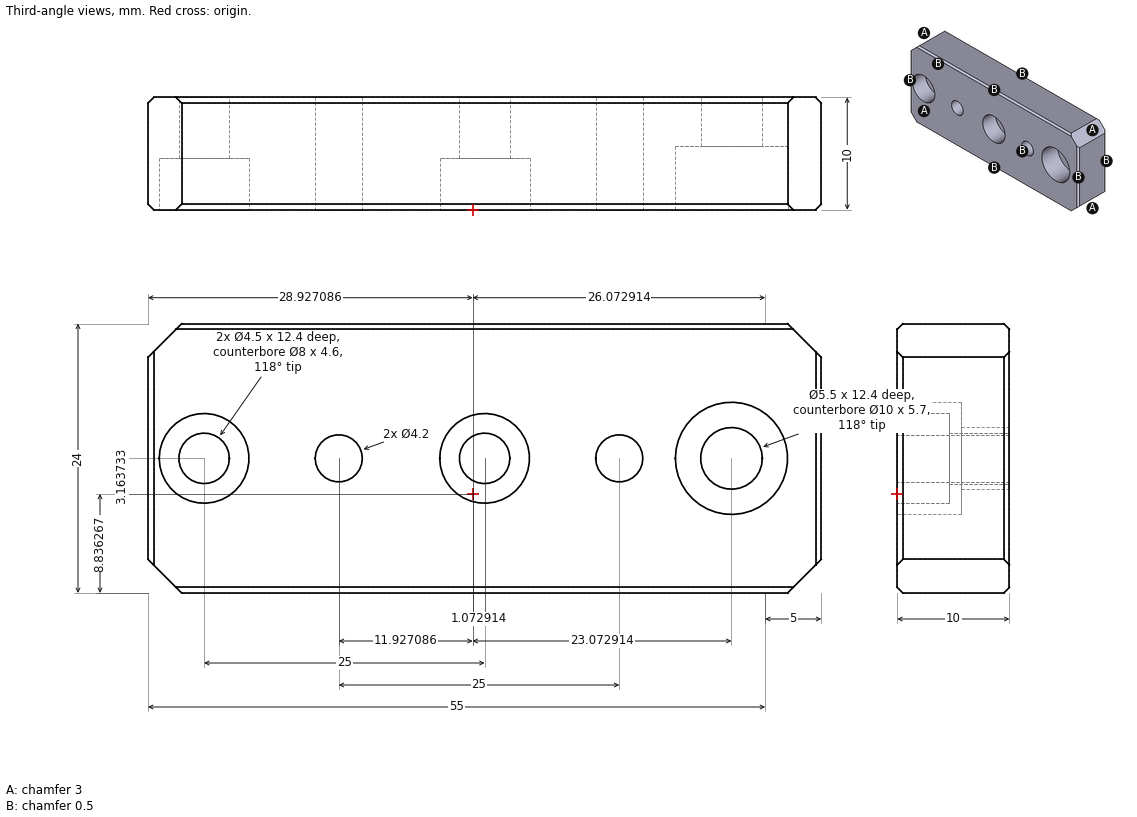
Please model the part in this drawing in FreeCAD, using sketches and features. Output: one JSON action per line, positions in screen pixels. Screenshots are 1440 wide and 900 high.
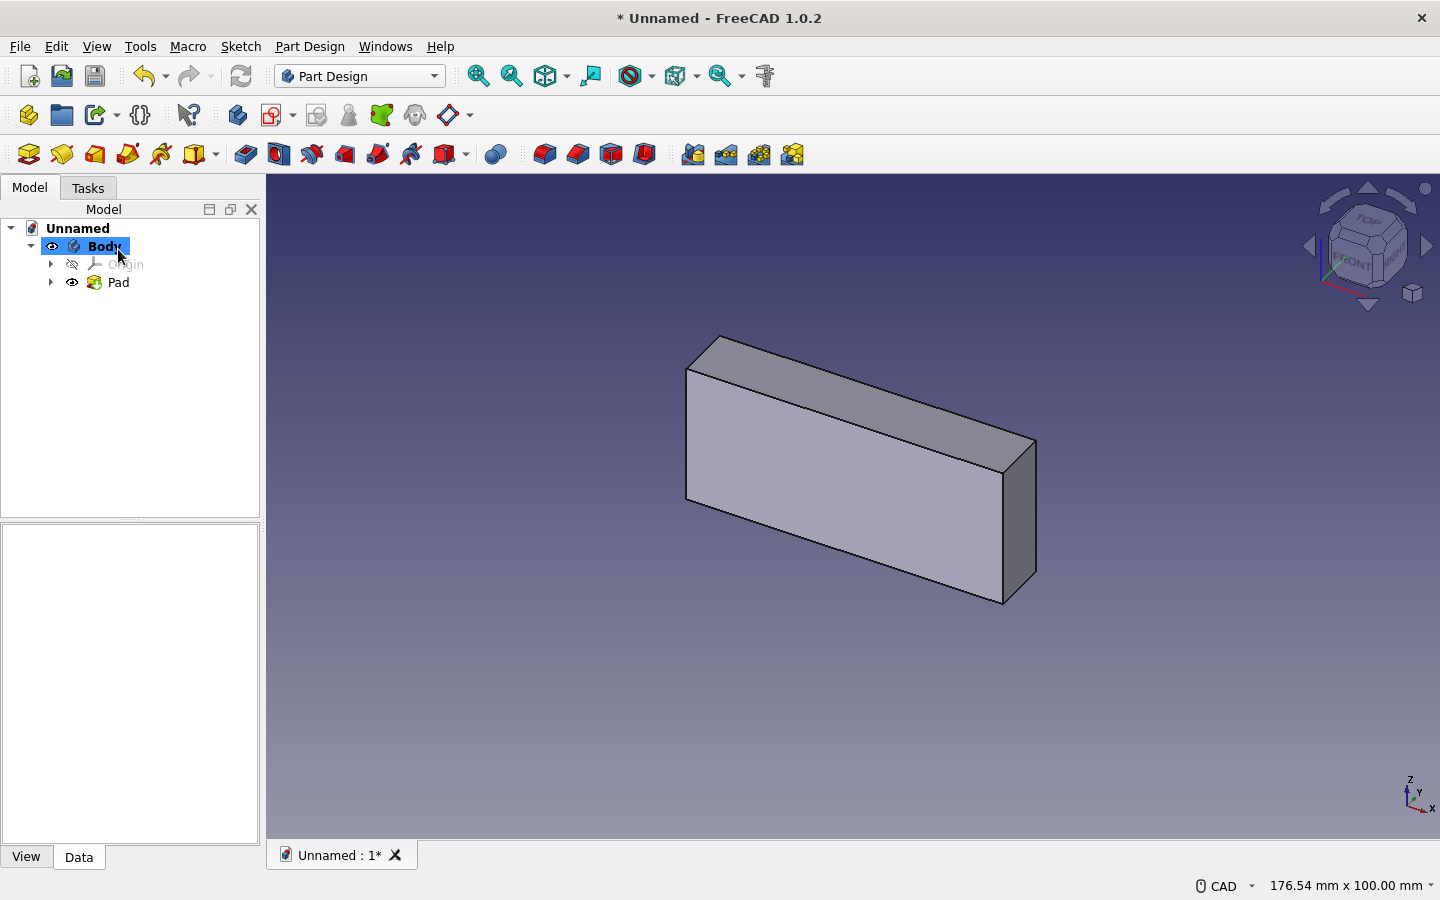
{"action": "key", "text": "v f"}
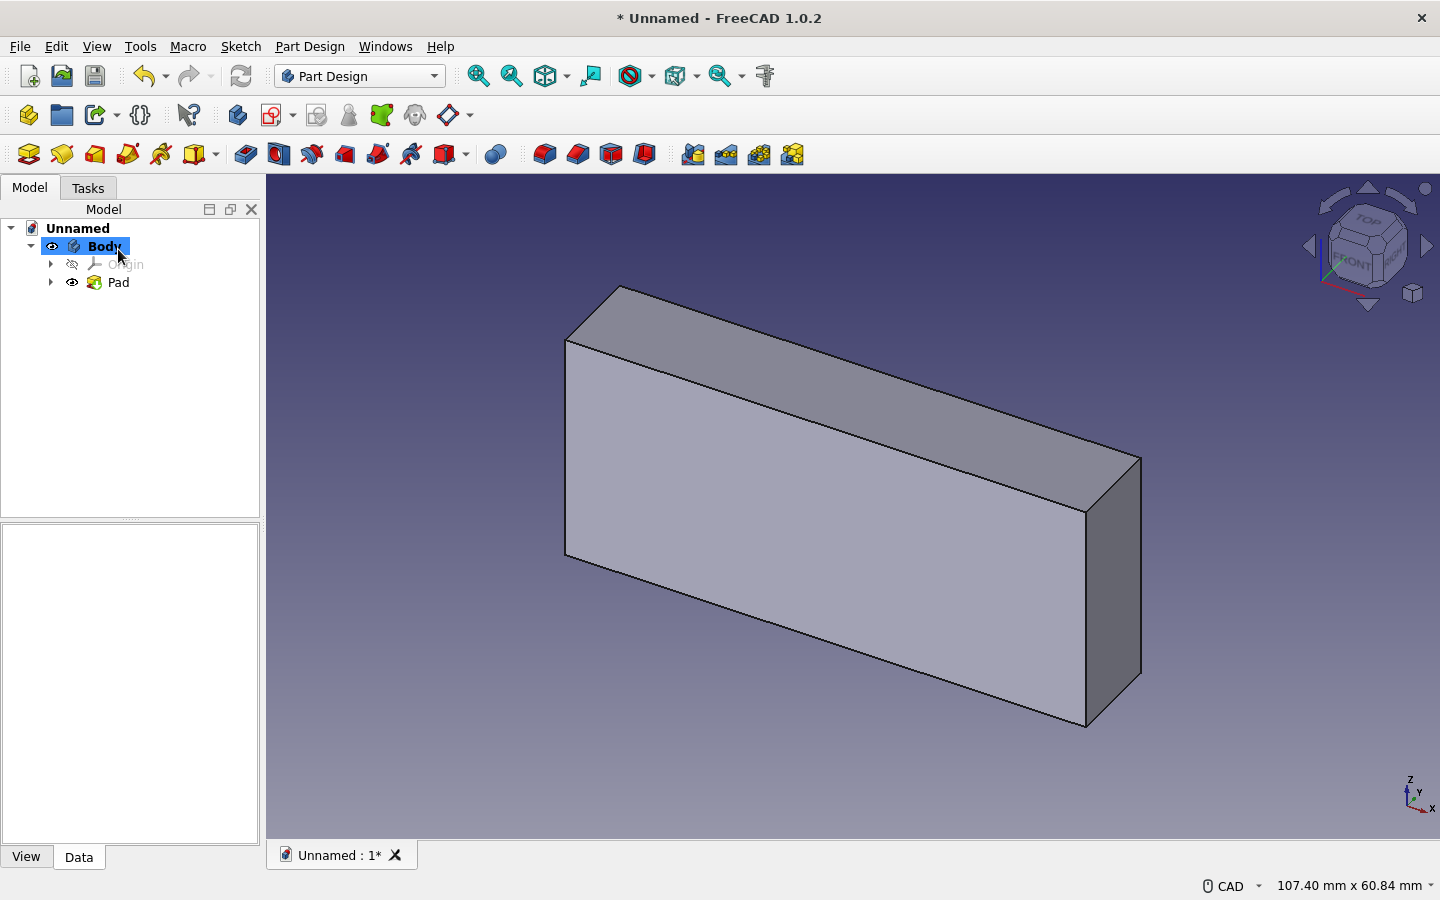
{"action": "left_click", "coordinate": [270, 116]}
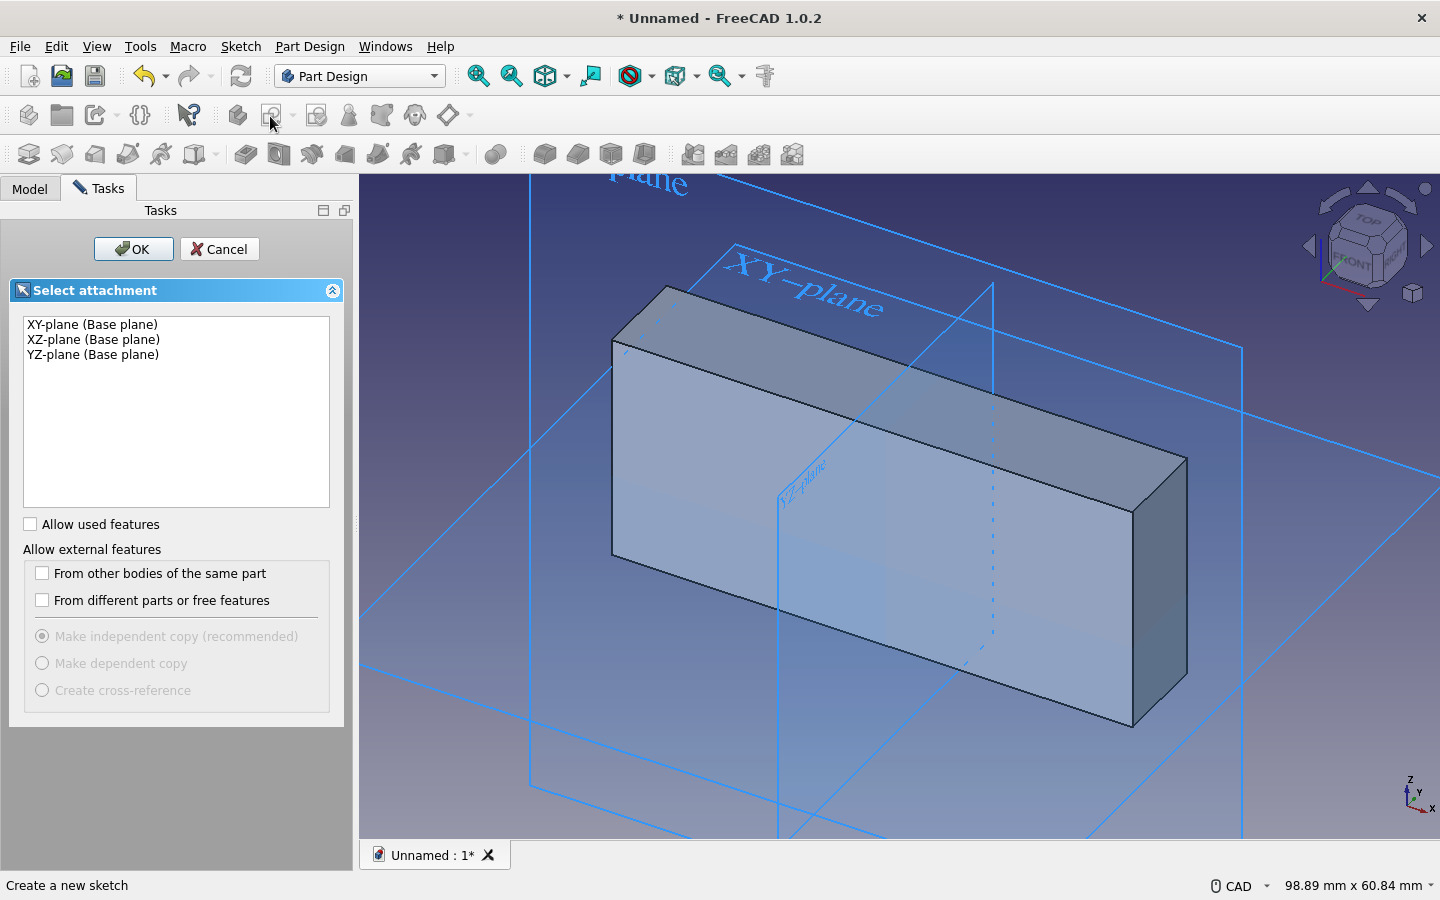
{"action": "left_click", "coordinate": [84, 340]}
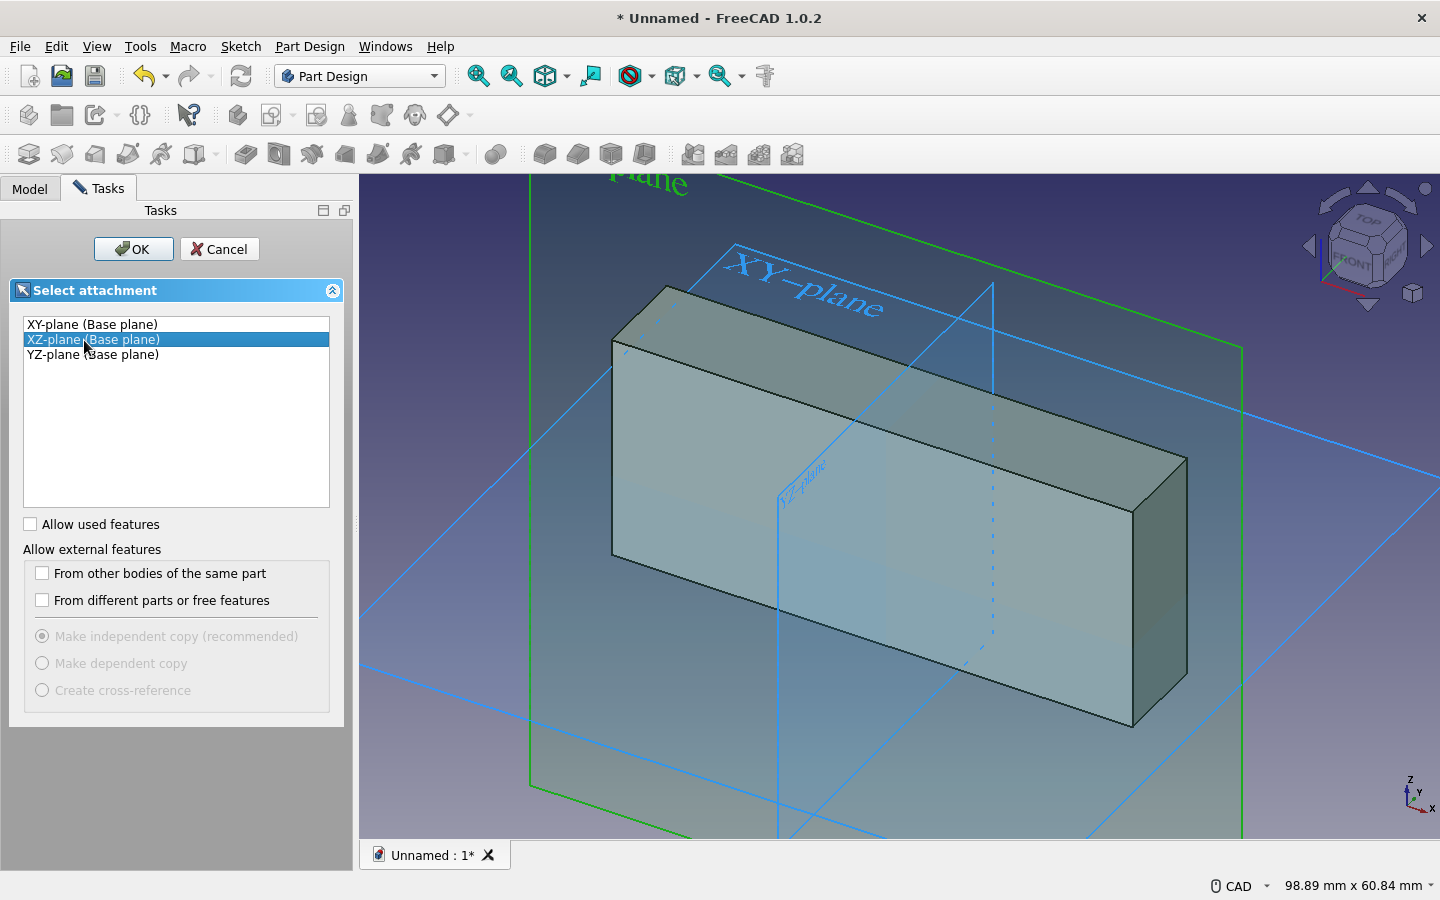
{"action": "left_click", "coordinate": [134, 249]}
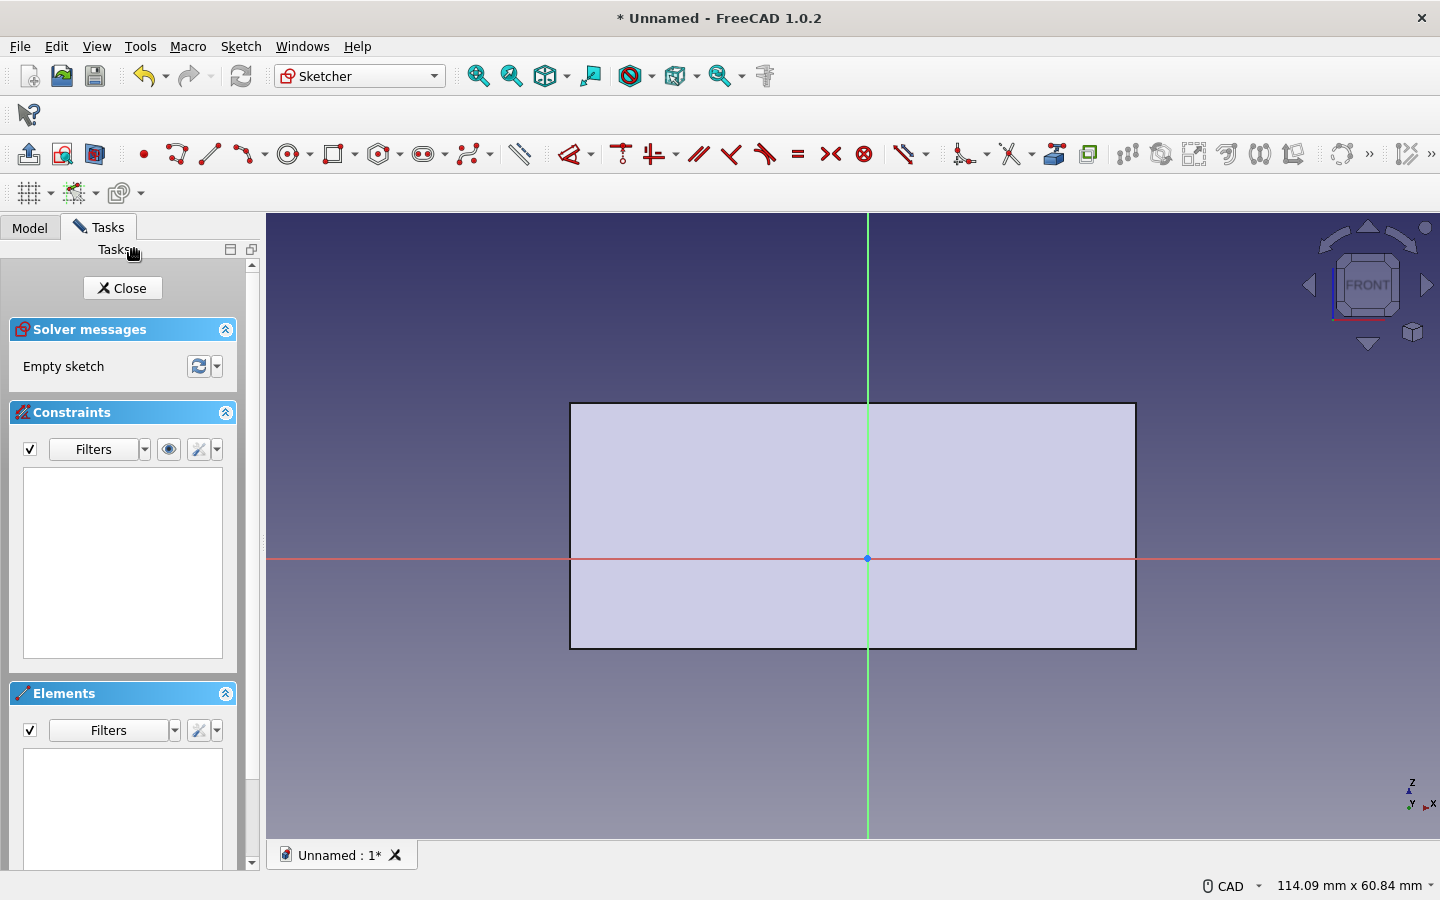
{"action": "scroll", "coordinate": [722, 535], "scroll_direction": "up", "scroll_amount": 4}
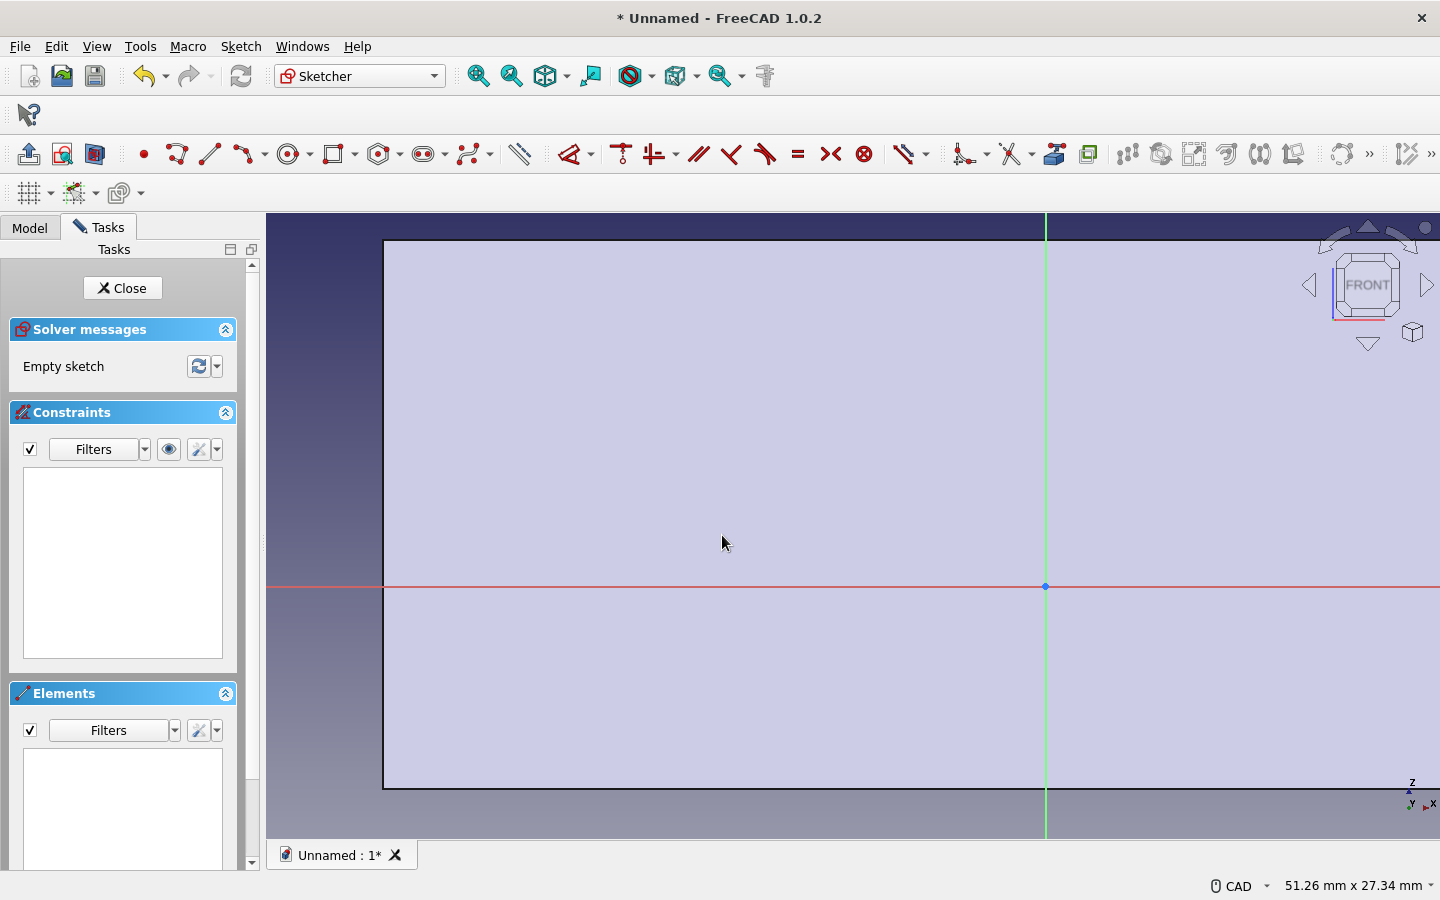
{"action": "key", "text": "g c"}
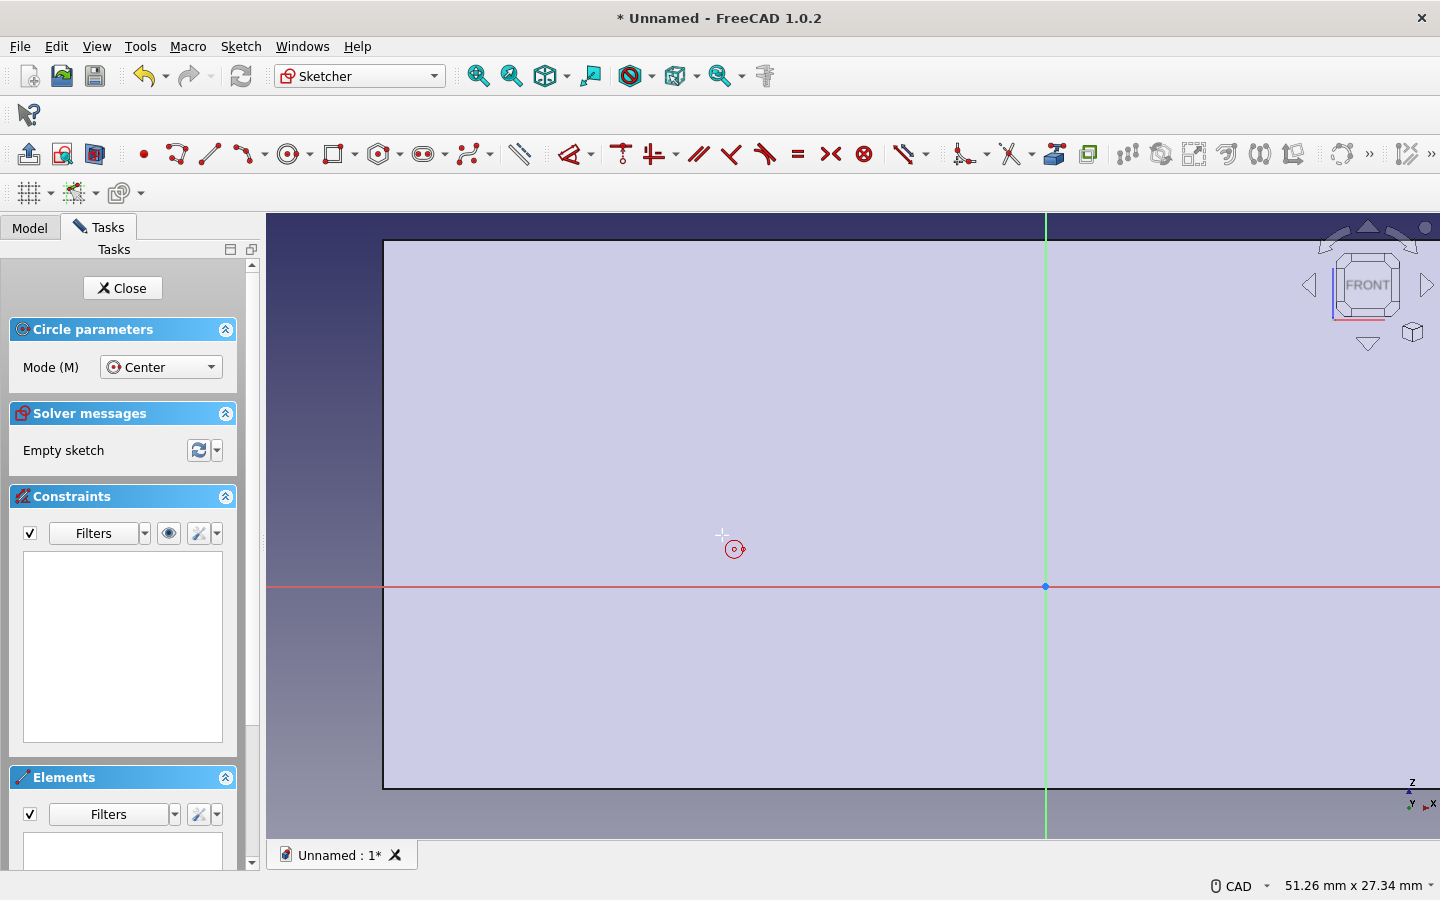
{"action": "left_click", "coordinate": [498, 514]}
{"action": "left_click", "coordinate": [534, 478]}